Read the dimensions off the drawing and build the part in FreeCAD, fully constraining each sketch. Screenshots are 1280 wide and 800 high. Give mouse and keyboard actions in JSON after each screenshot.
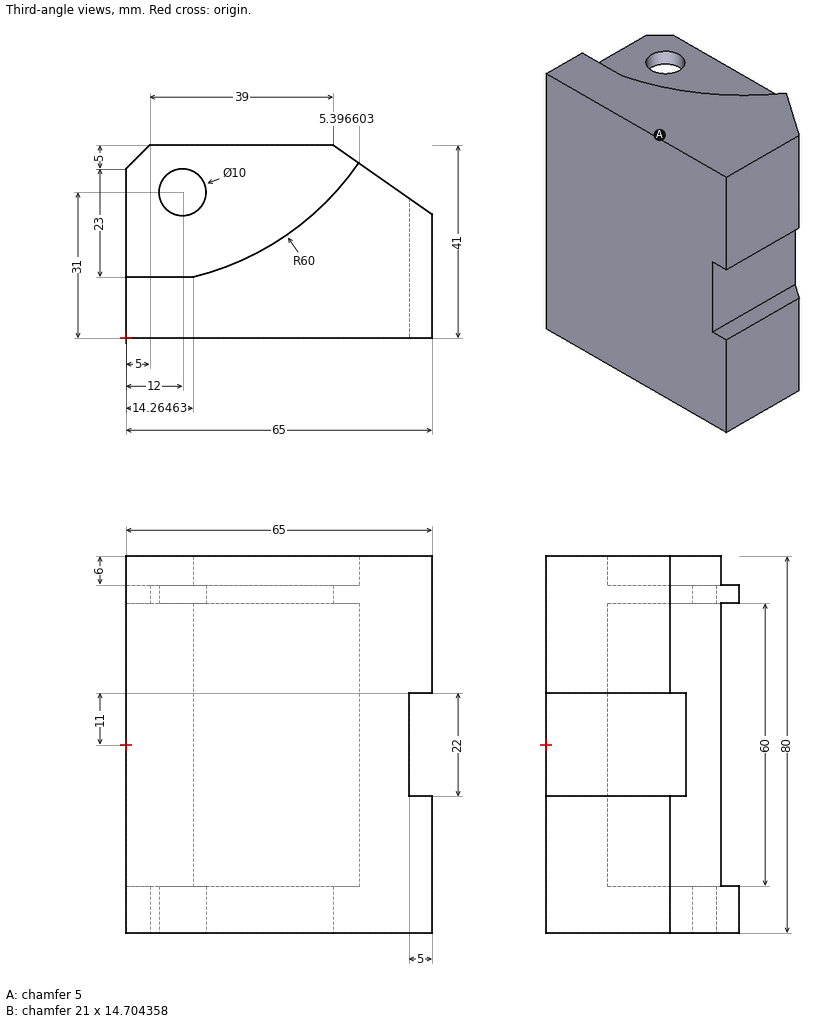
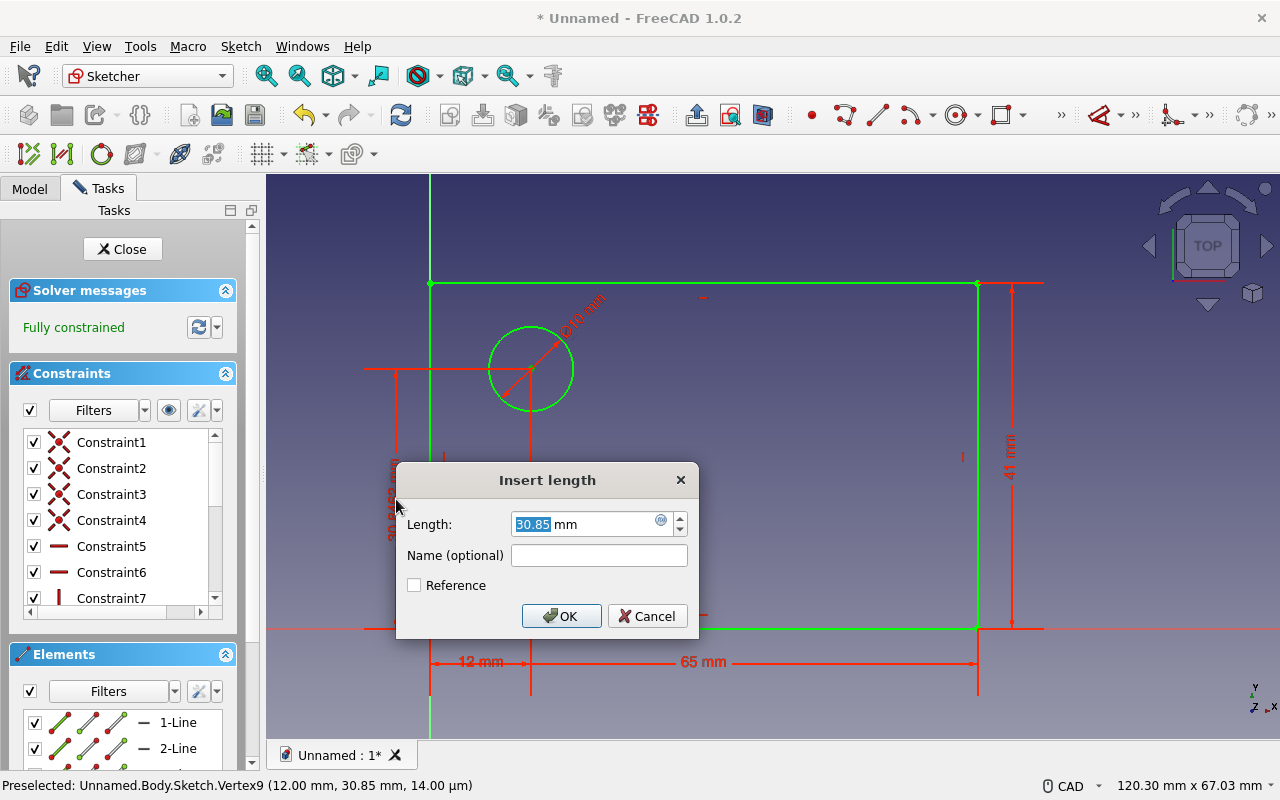
{"action": "type", "text": "31"}
{"action": "key", "text": "Return"}
{"action": "key", "text": "Escape"}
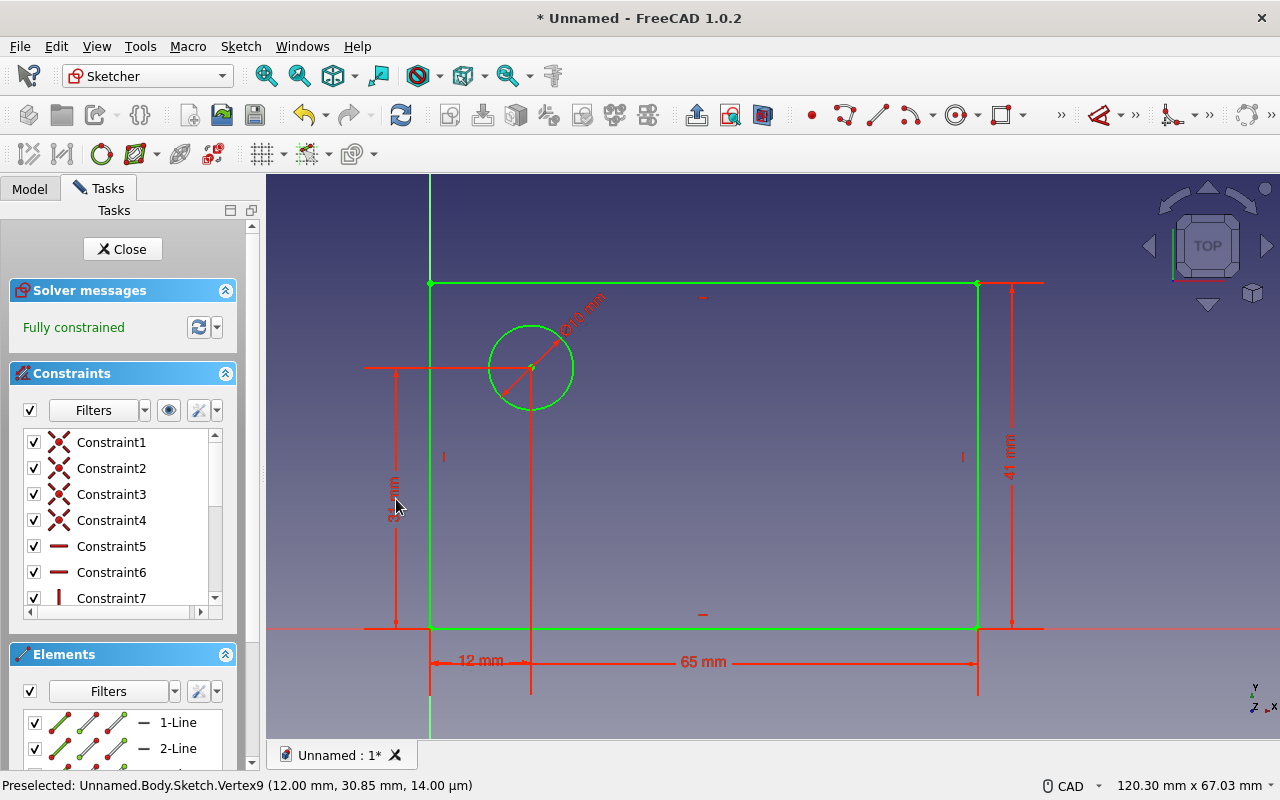
{"action": "left_click", "coordinate": [123, 249]}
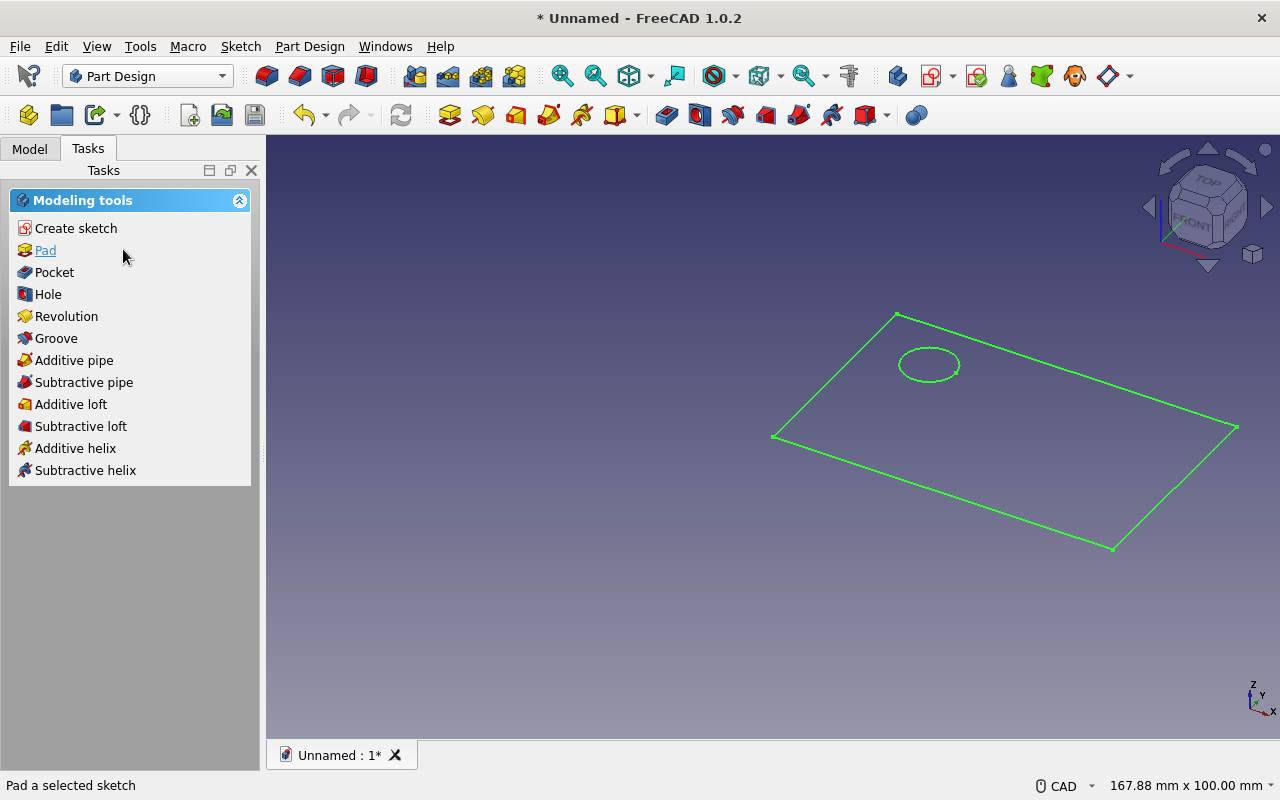
{"action": "left_click", "coordinate": [450, 116]}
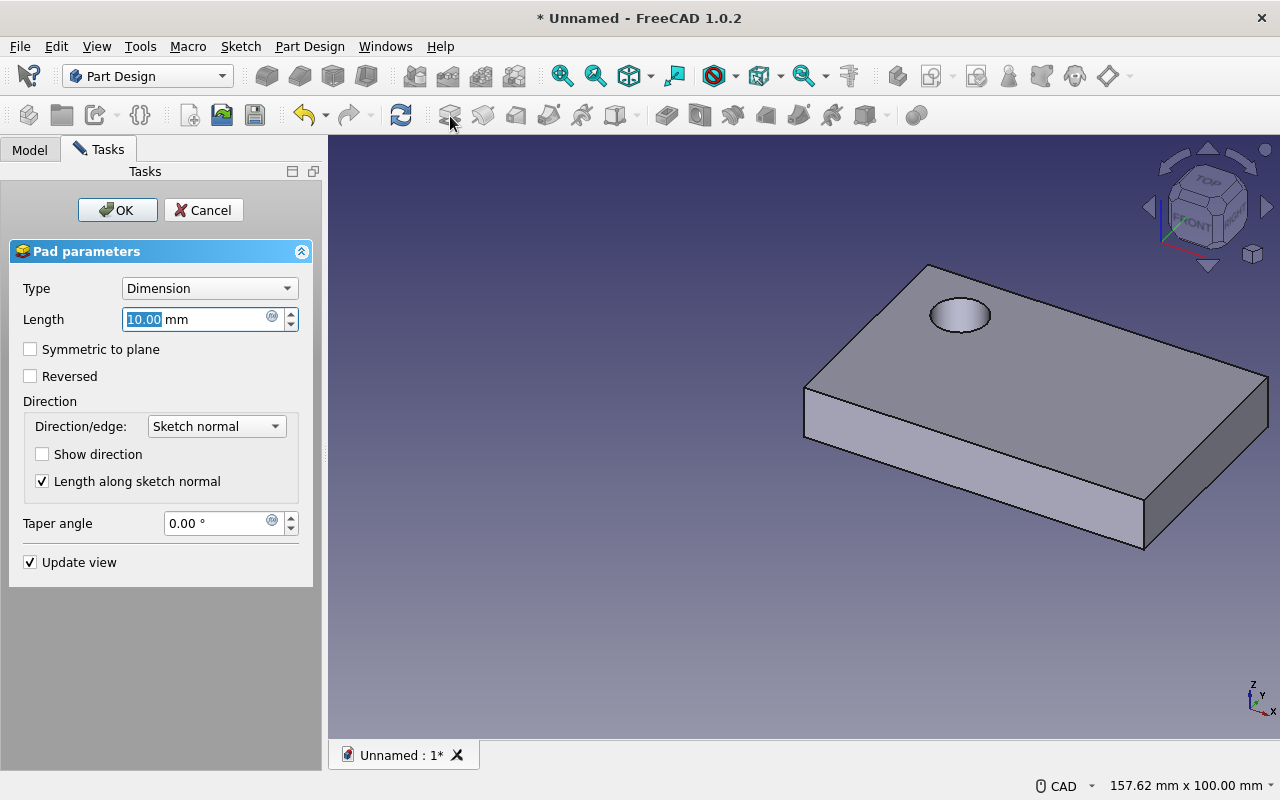
{"action": "type", "text": "80"}
{"action": "key", "text": "Tab"}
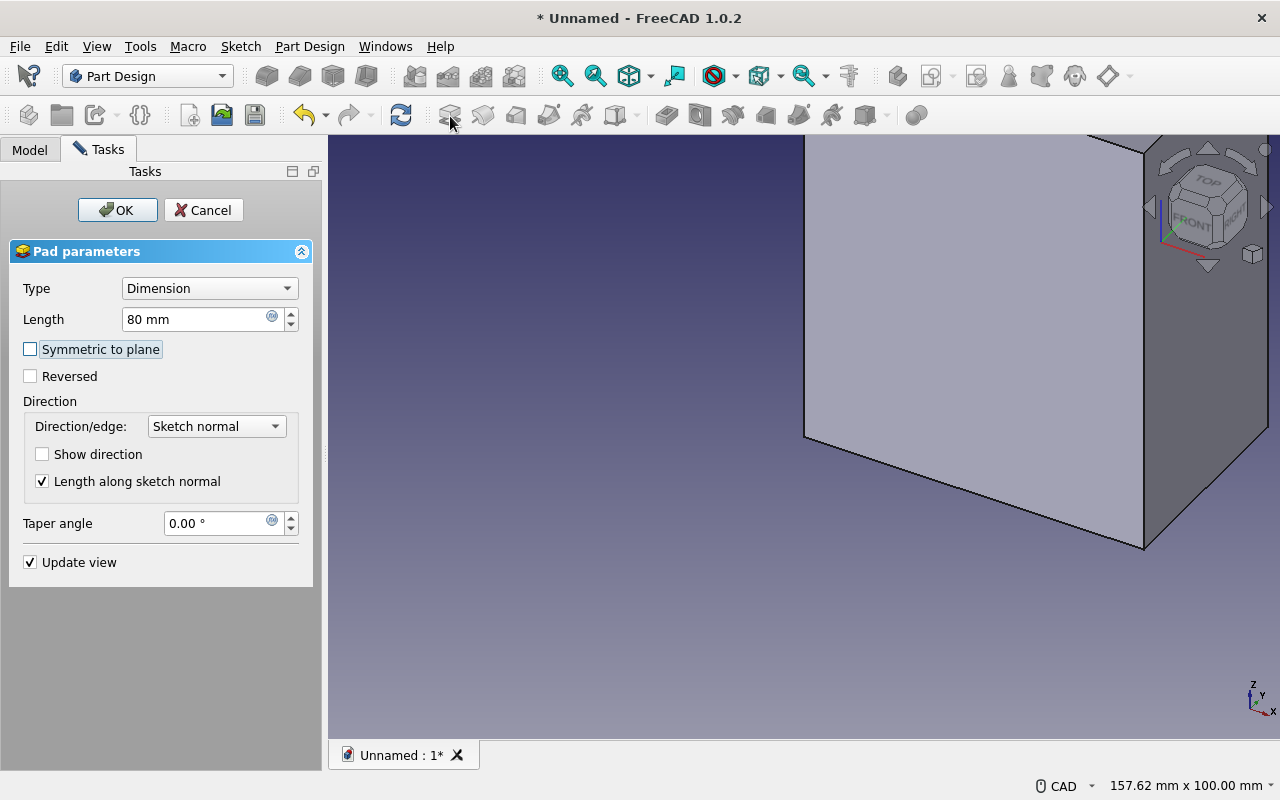
{"action": "left_click", "coordinate": [31, 349]}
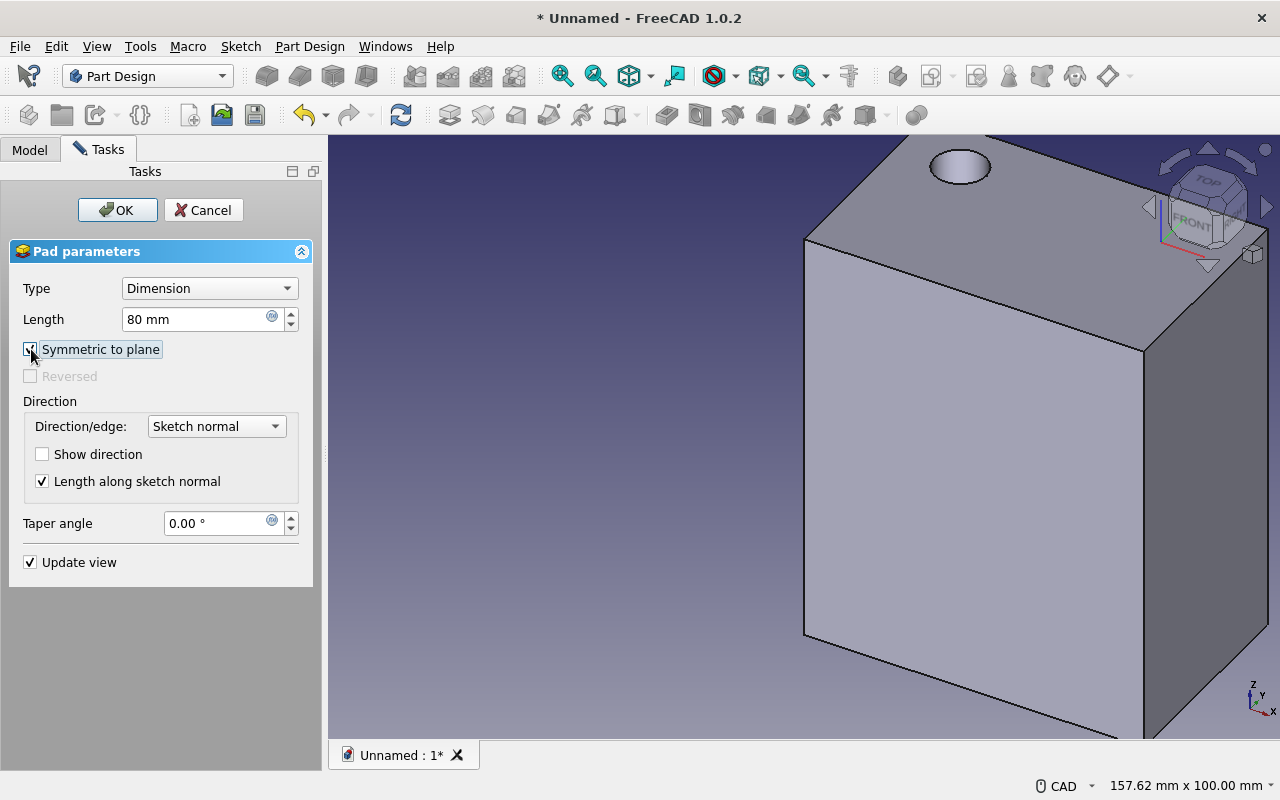
{"action": "left_click", "coordinate": [118, 210]}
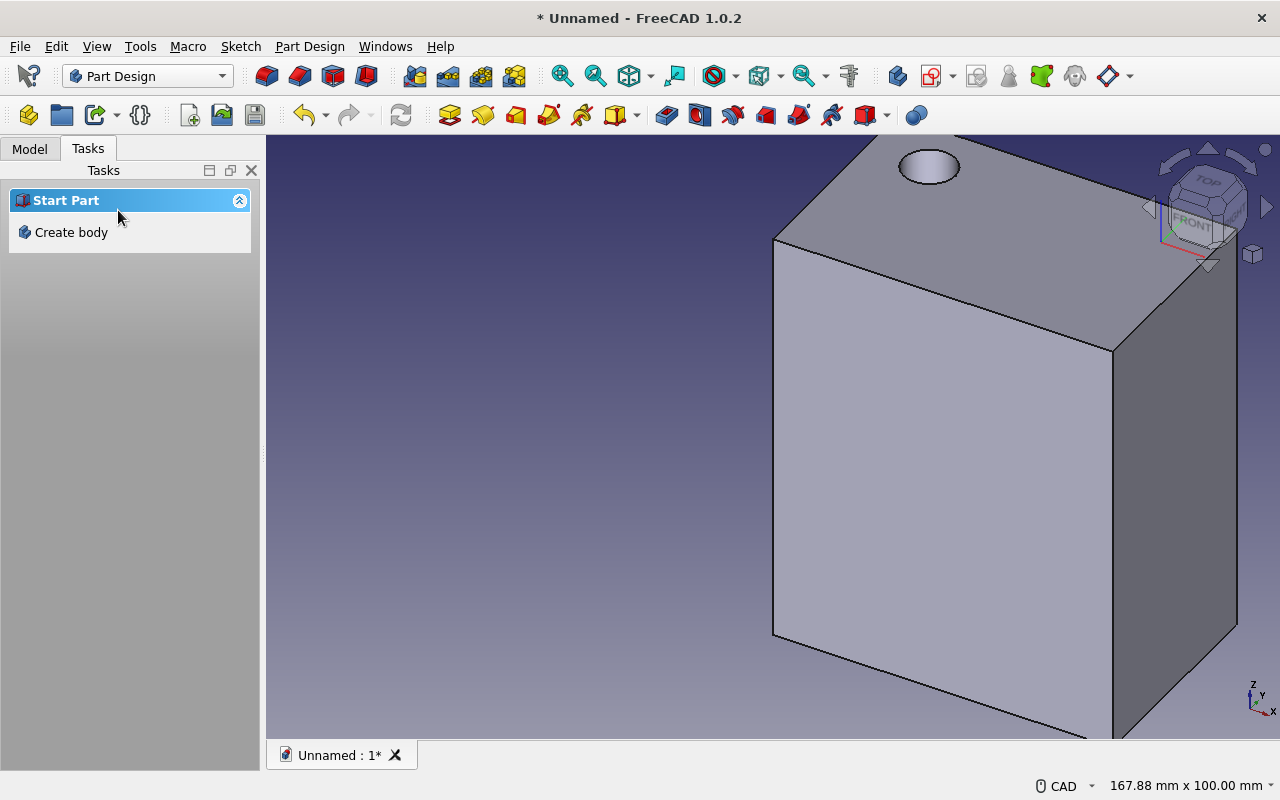
{"action": "key", "text": "v f"}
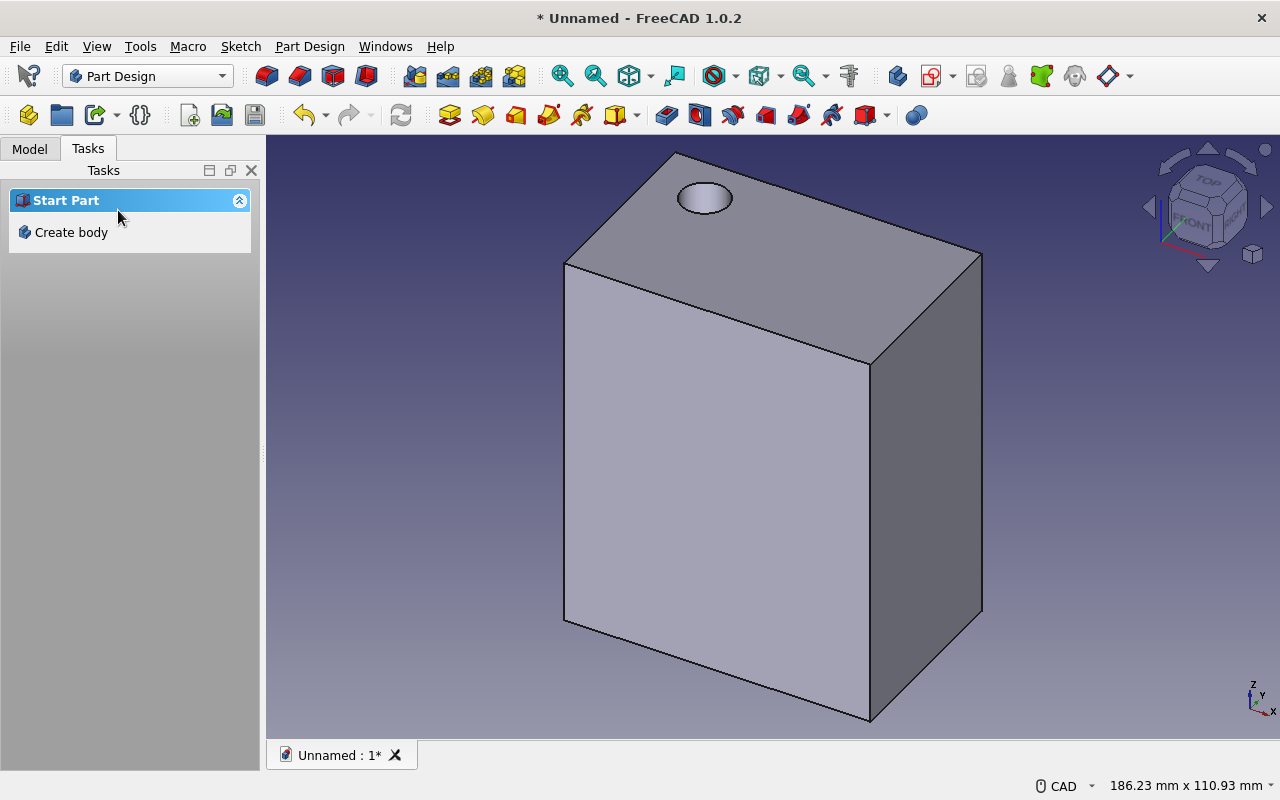
{"action": "key", "text": "0"}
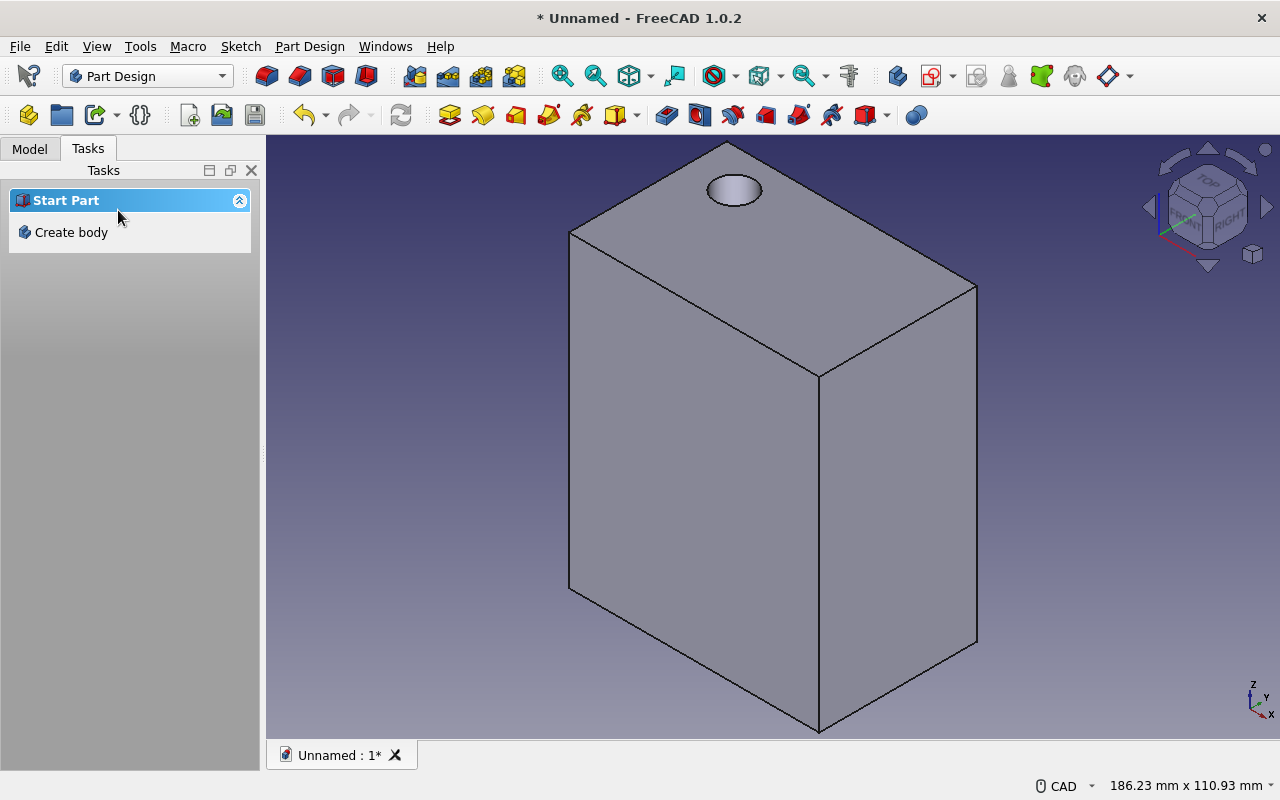
{"action": "key", "text": "2"}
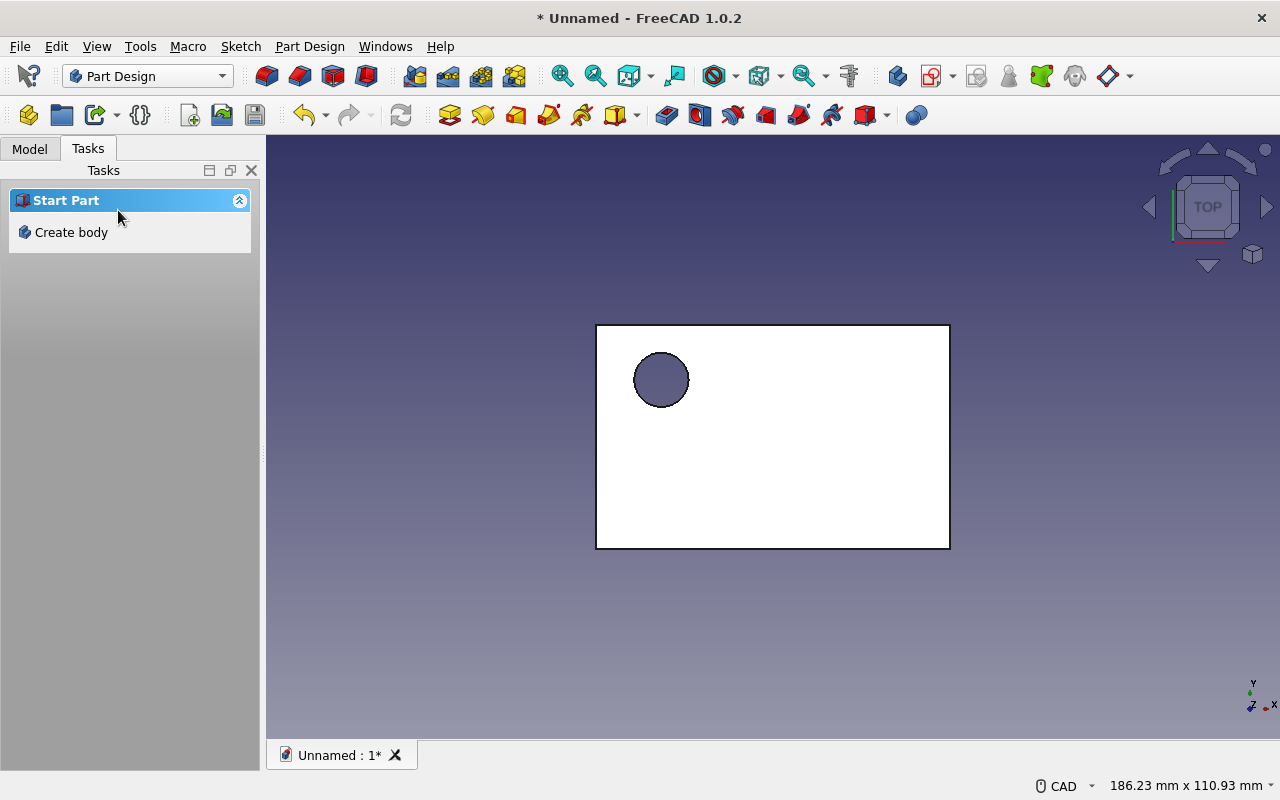
{"action": "left_click", "coordinate": [563, 76]}